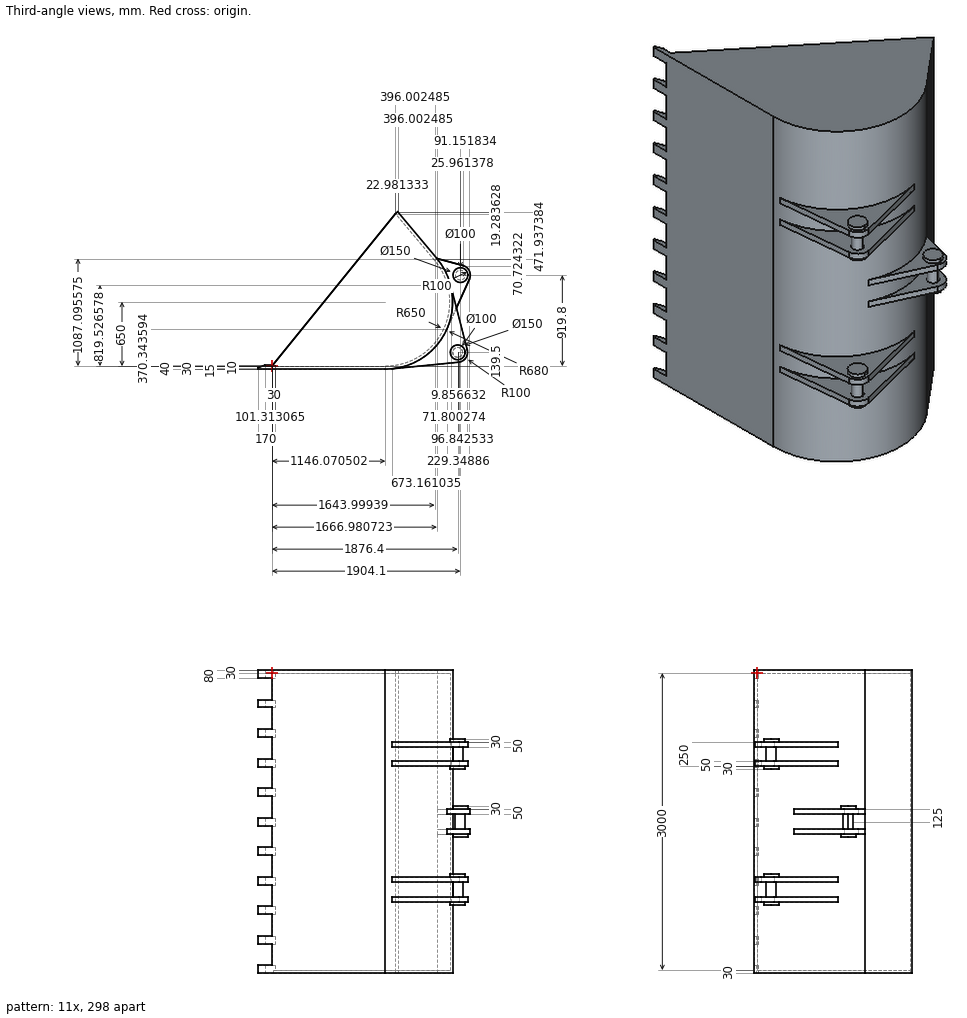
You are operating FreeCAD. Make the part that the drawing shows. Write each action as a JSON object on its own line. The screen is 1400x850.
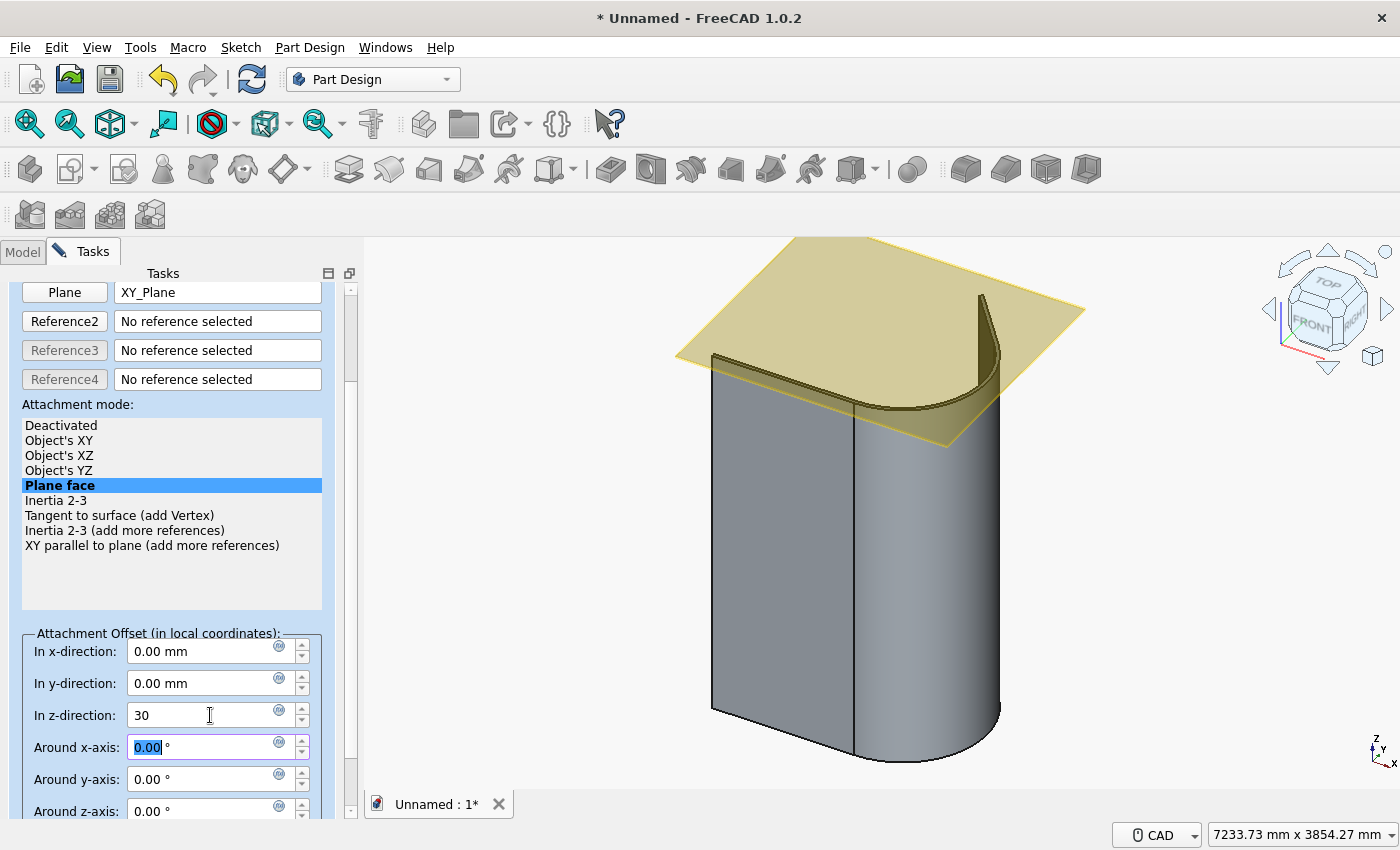
{"action": "scroll", "coordinate": [351, 550], "scroll_direction": "up", "scroll_amount": 3}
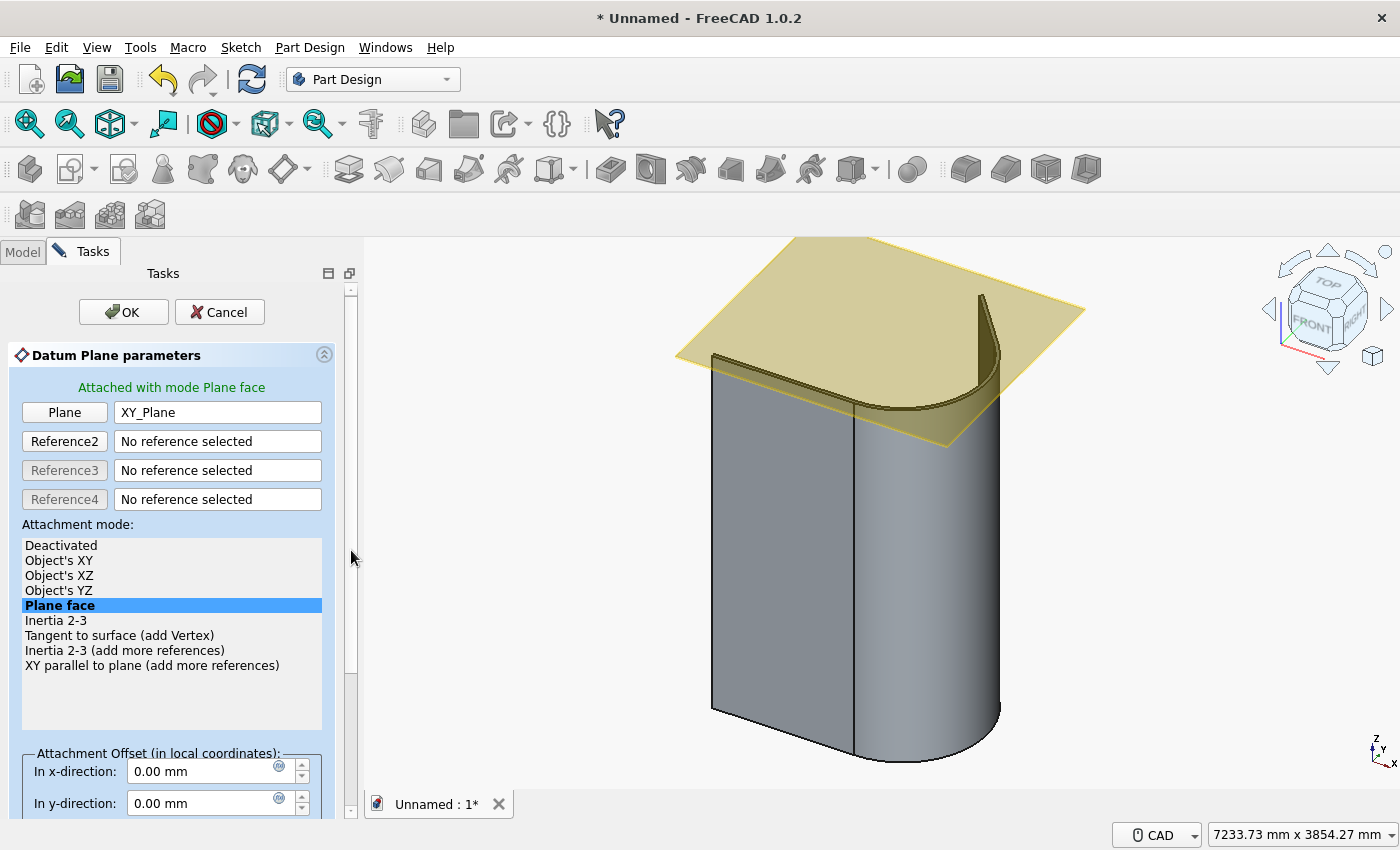
{"action": "left_click", "coordinate": [124, 312]}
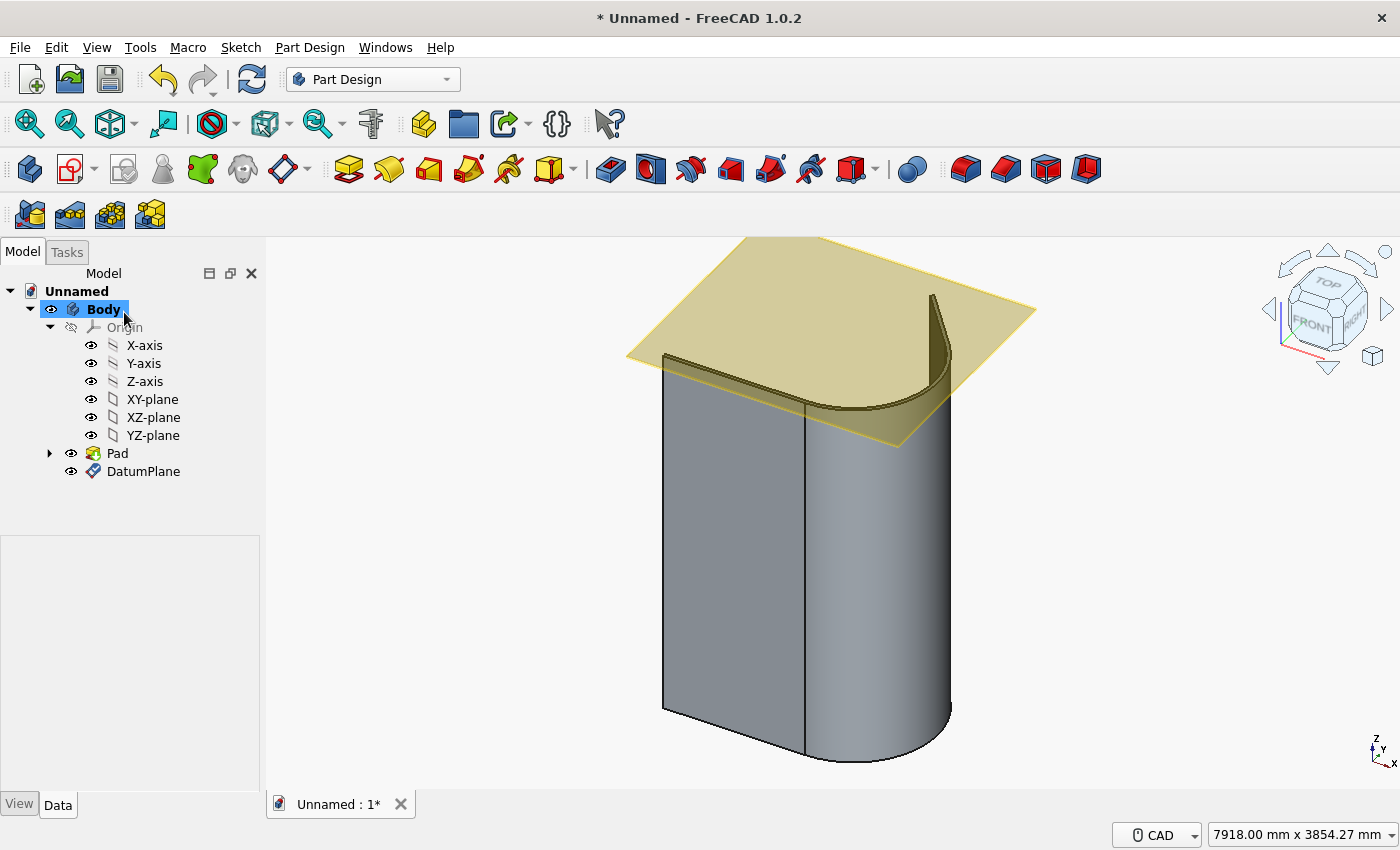
{"action": "left_click", "coordinate": [116, 471]}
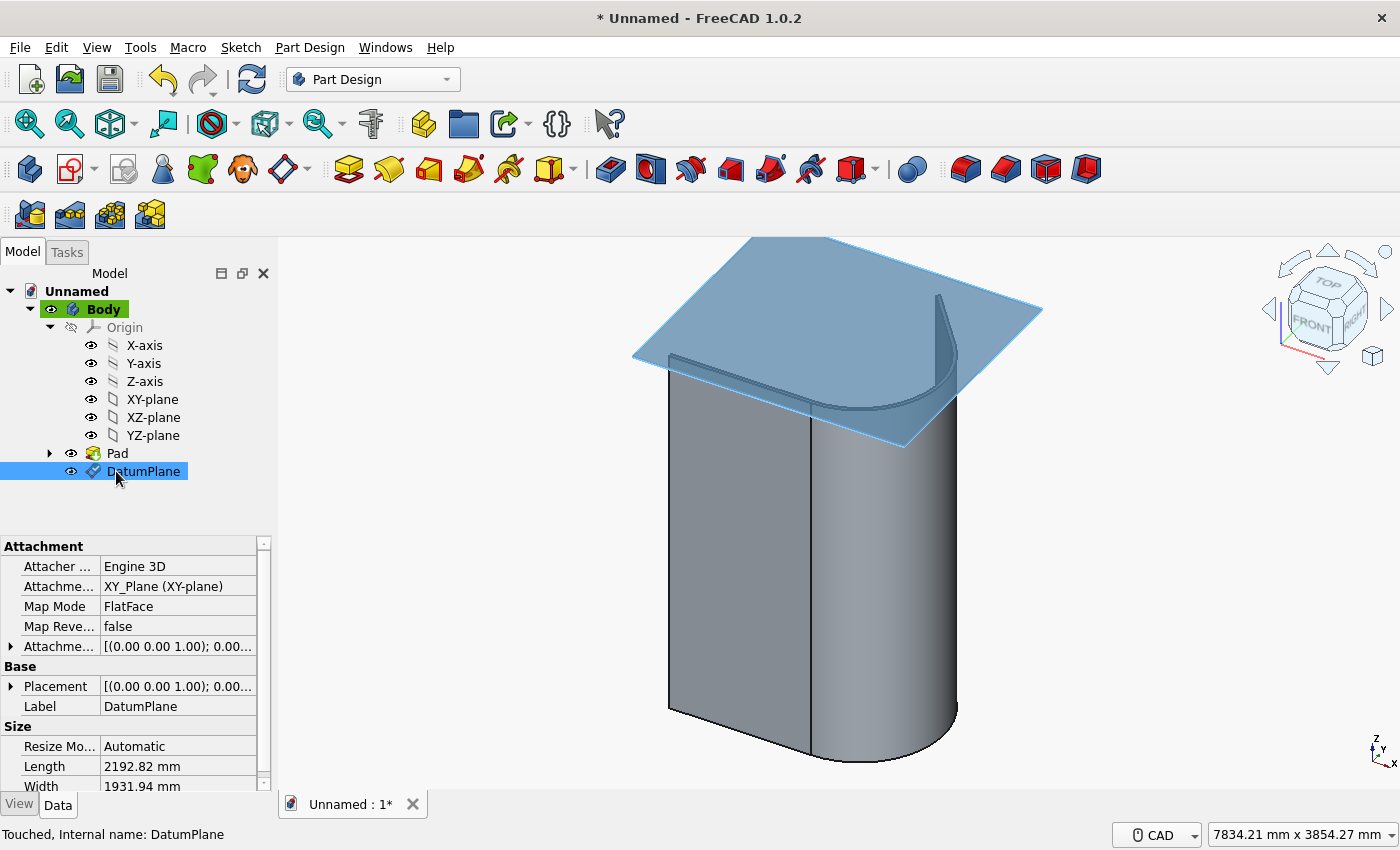
{"action": "left_click", "coordinate": [70, 170]}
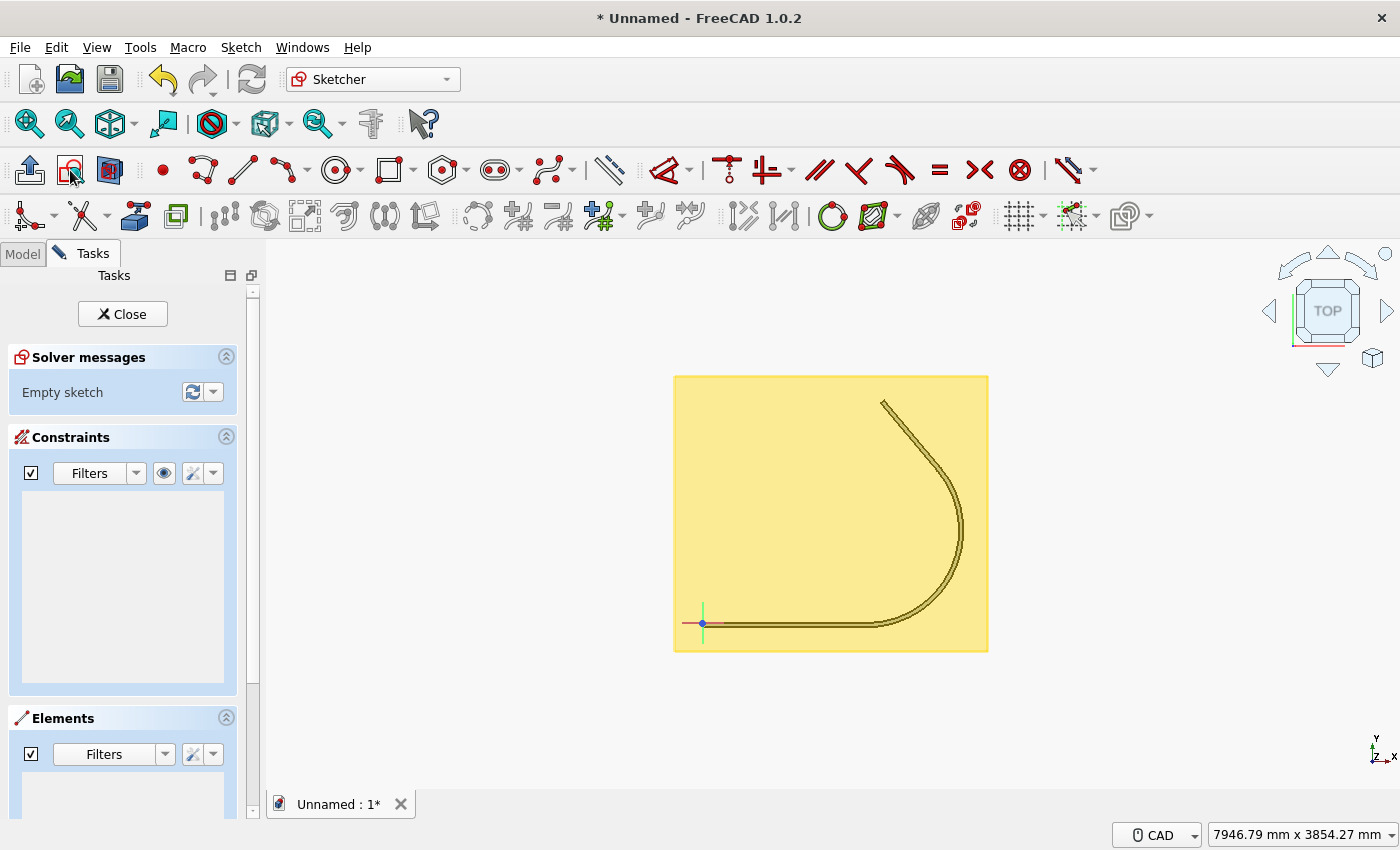
{"action": "scroll", "coordinate": [959, 514], "scroll_direction": "up", "scroll_amount": 2}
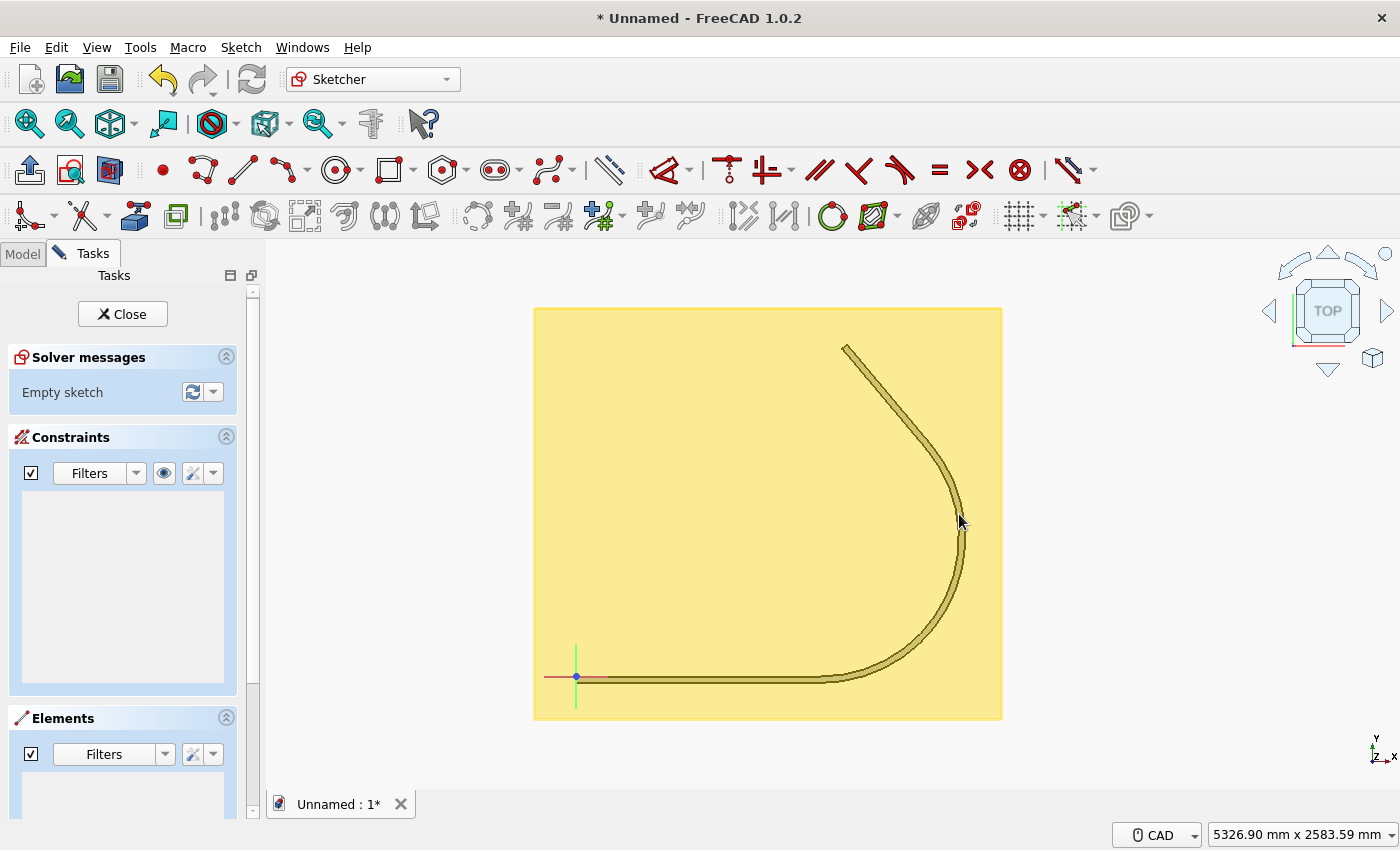
{"action": "key", "text": "g m"}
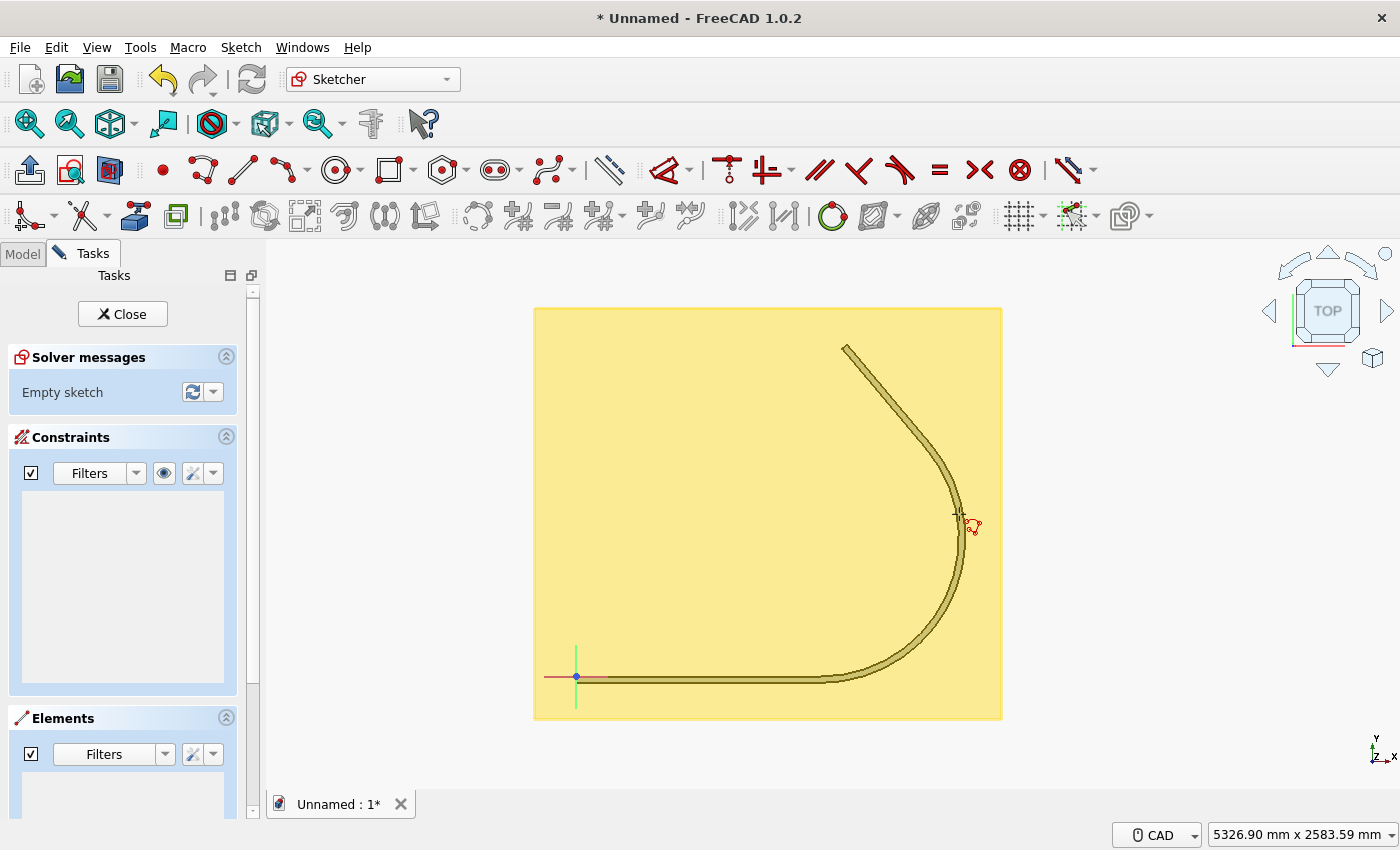
{"action": "left_click", "coordinate": [931, 445]}
{"action": "left_click", "coordinate": [847, 345]}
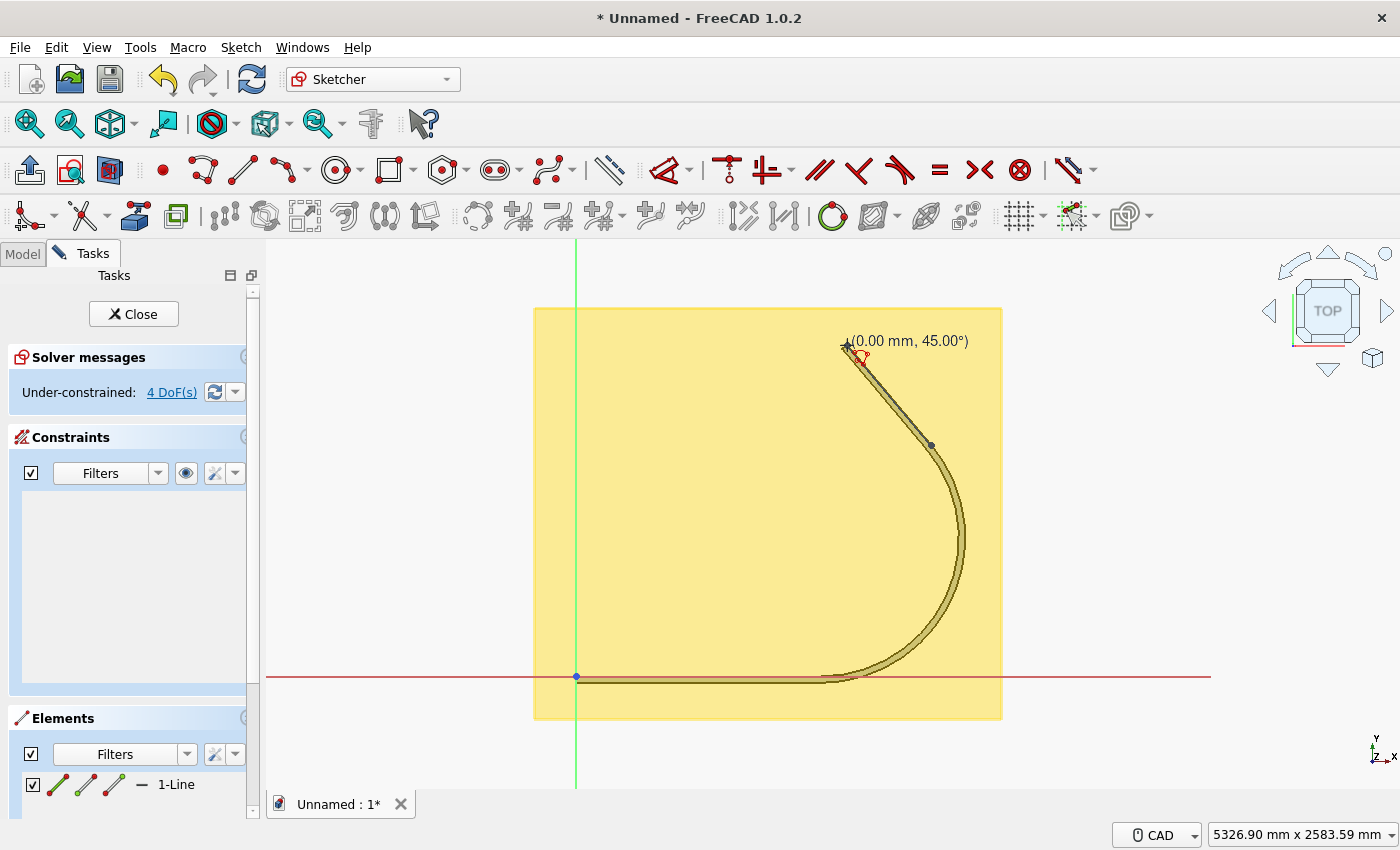
{"action": "scroll", "coordinate": [842, 349], "scroll_direction": "up", "scroll_amount": 5}